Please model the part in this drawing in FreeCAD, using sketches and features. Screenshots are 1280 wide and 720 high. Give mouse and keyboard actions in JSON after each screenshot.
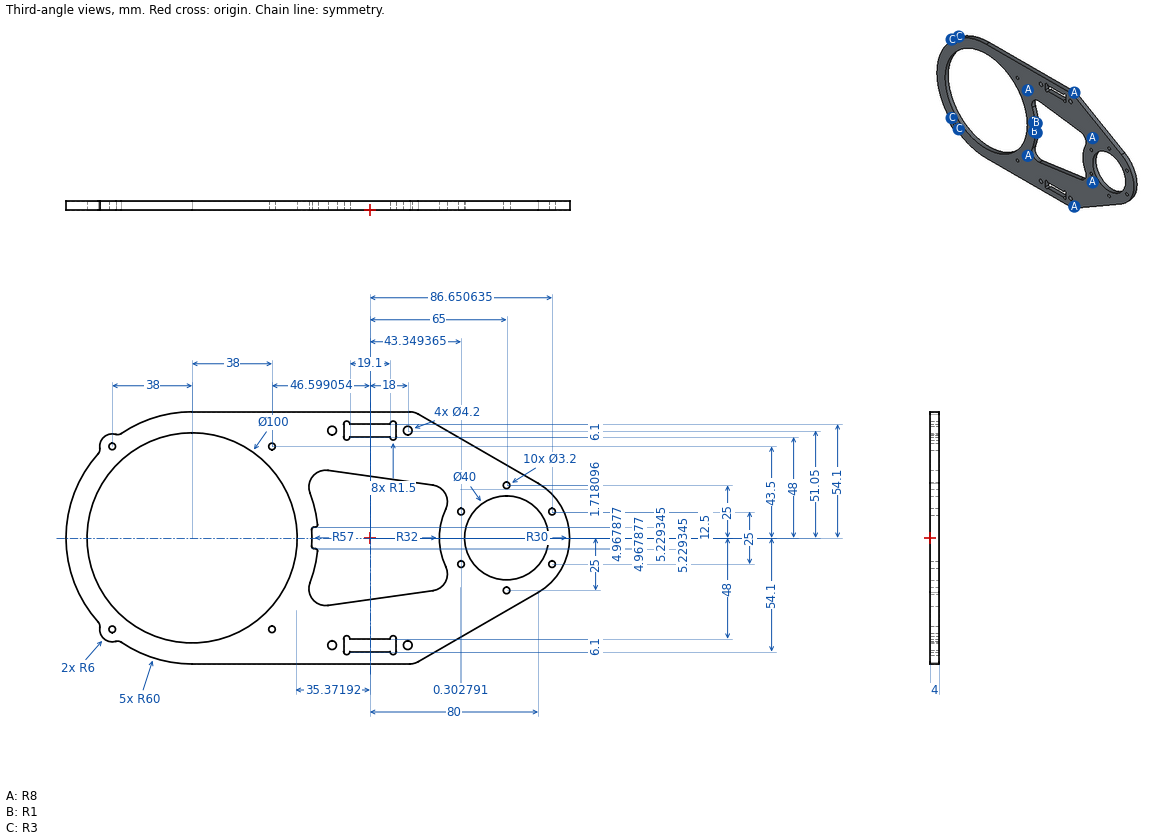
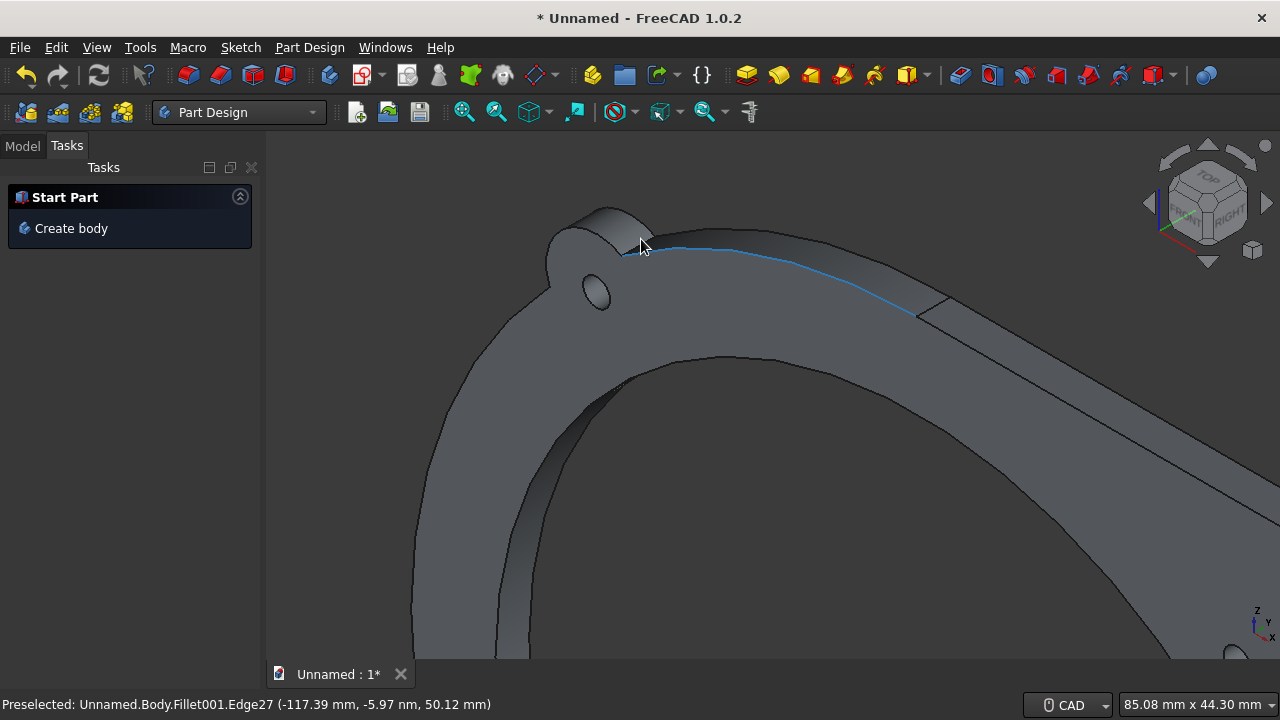
{"action": "left_click", "coordinate": [466, 112]}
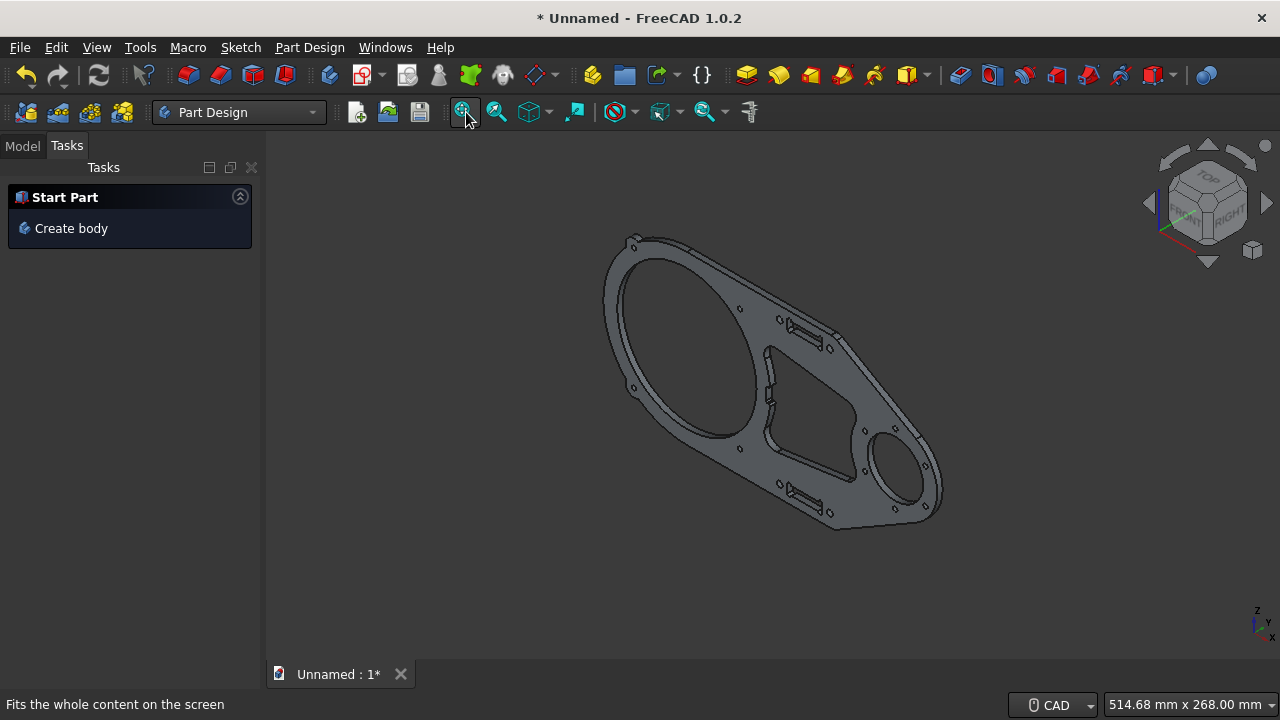
{"action": "key", "text": "2"}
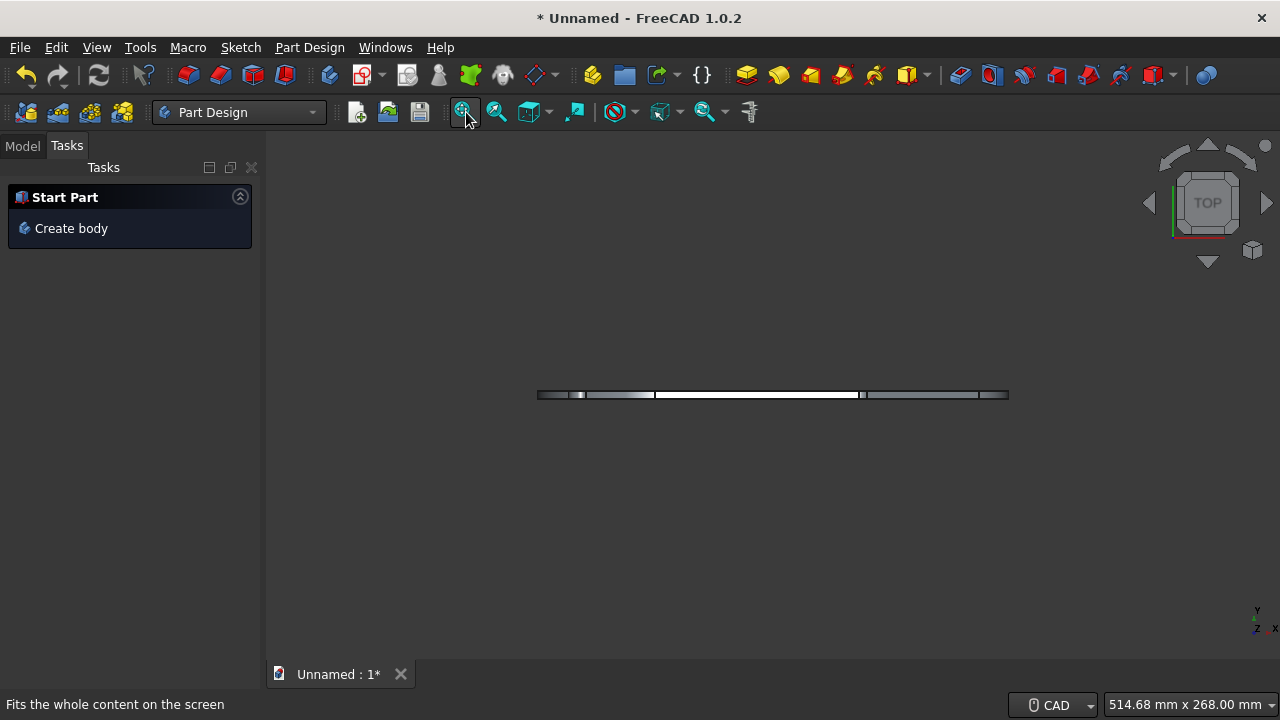
{"action": "scroll", "coordinate": [586, 394], "scroll_direction": "up", "scroll_amount": 9}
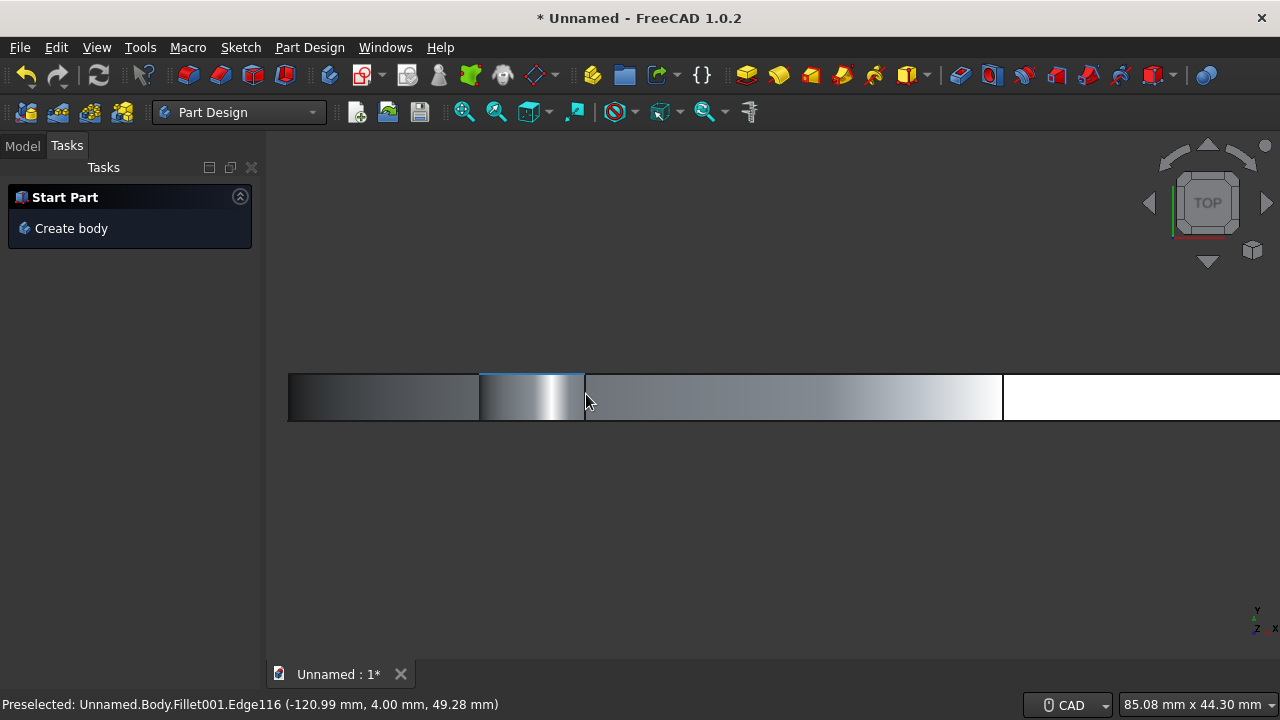
{"action": "left_click", "coordinate": [466, 112]}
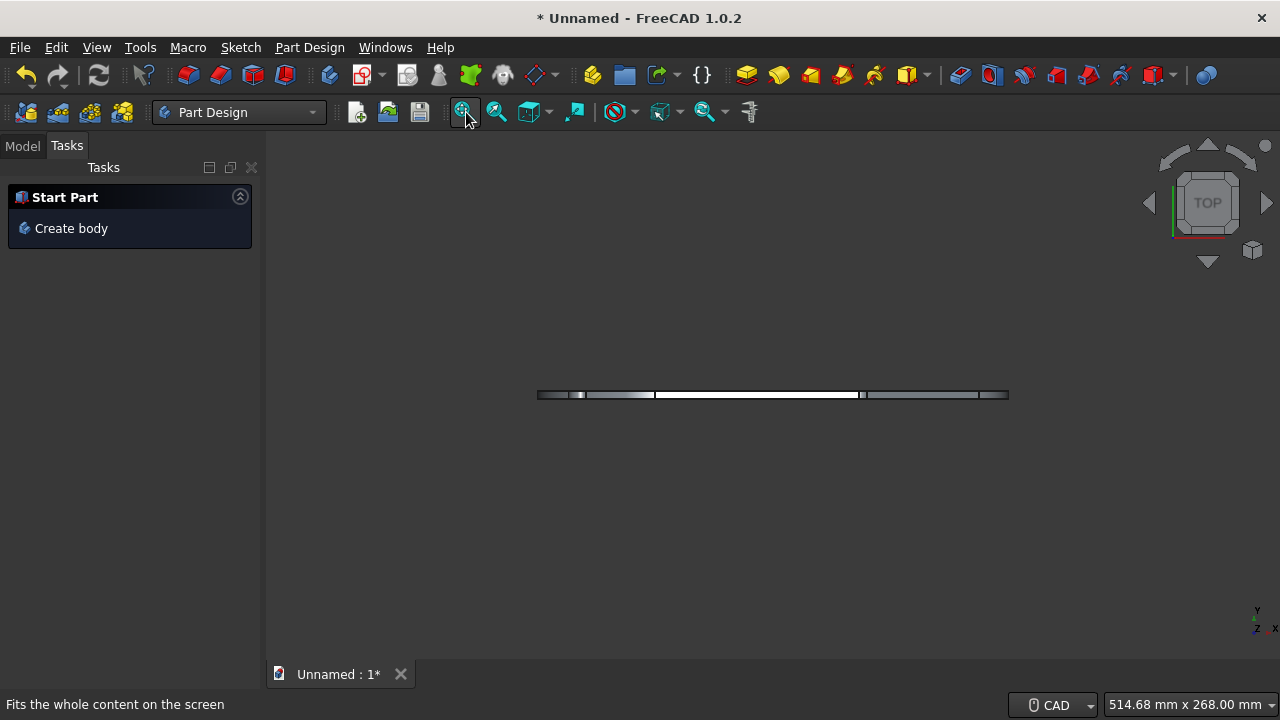
{"action": "key", "text": "0"}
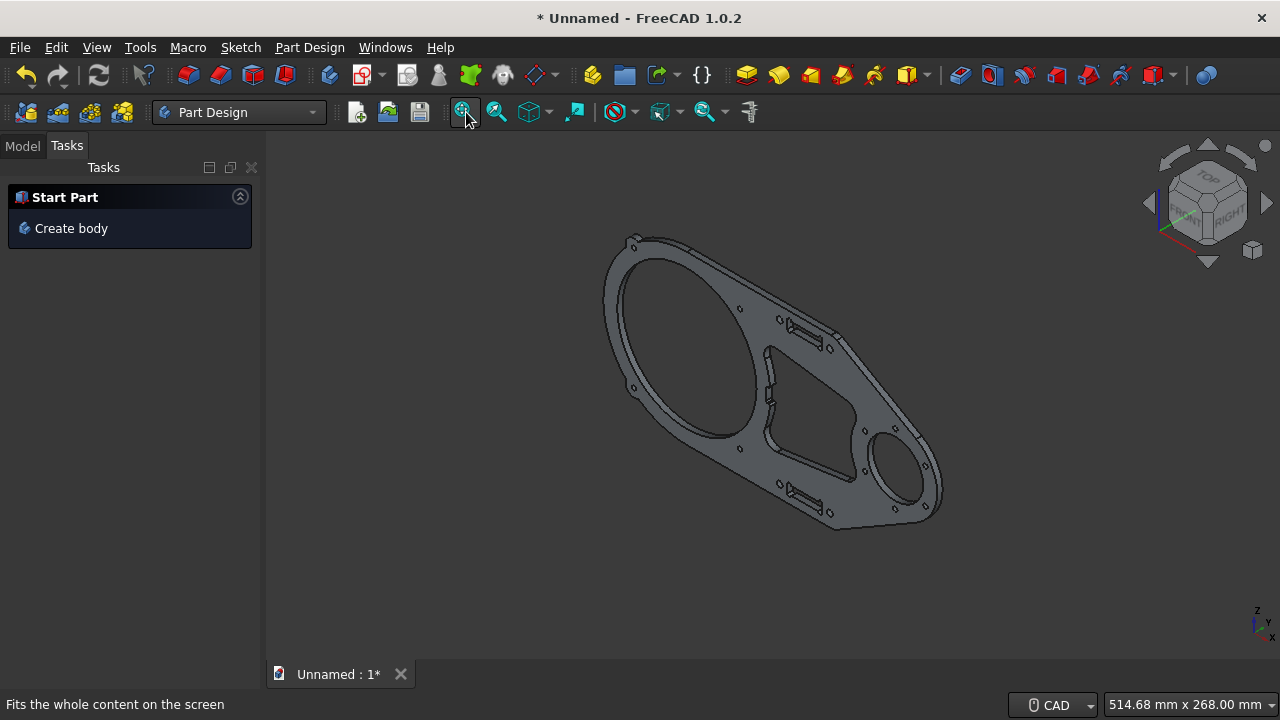
{"action": "scroll", "coordinate": [641, 239], "scroll_direction": "up", "scroll_amount": 9}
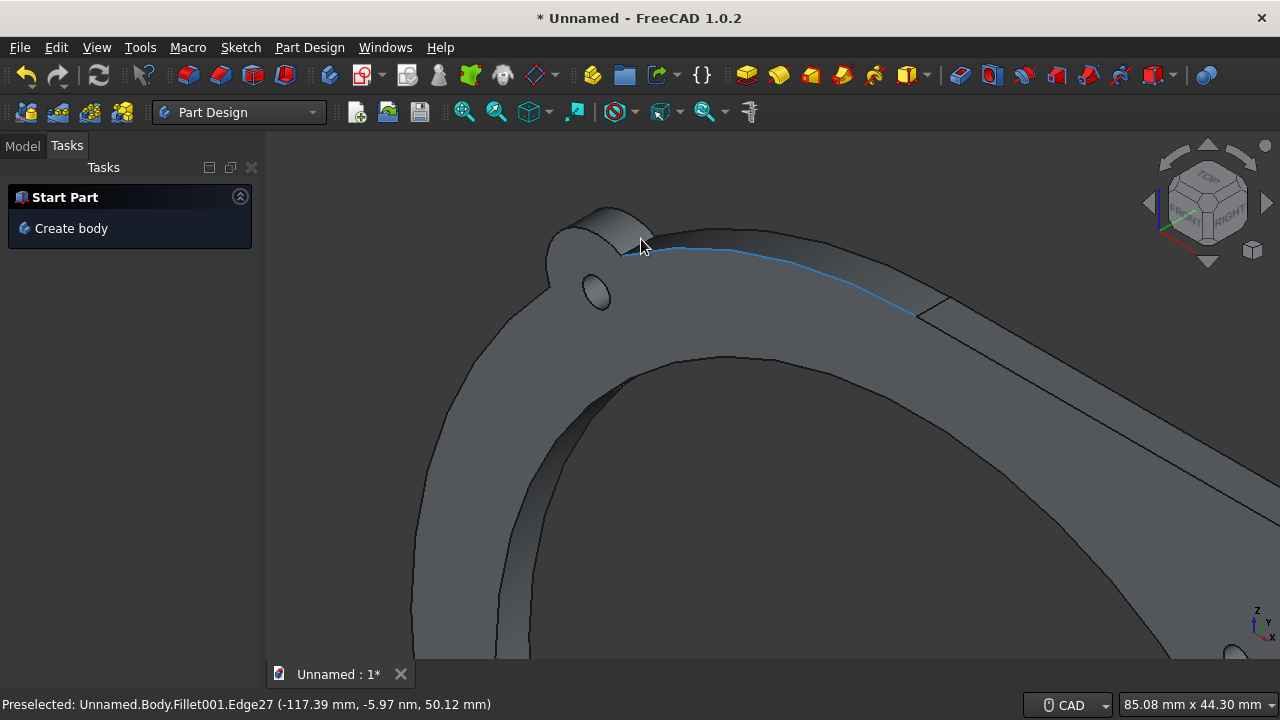
{"action": "key", "text": "v f"}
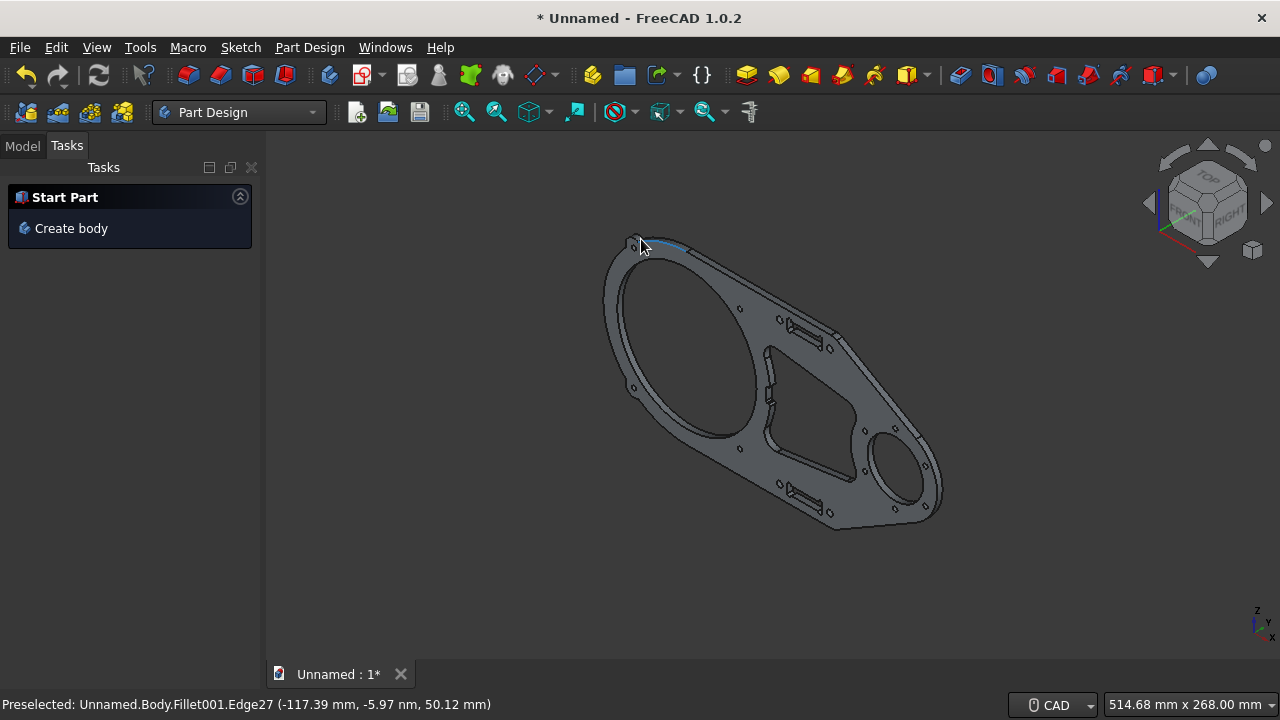
{"action": "key", "text": "1"}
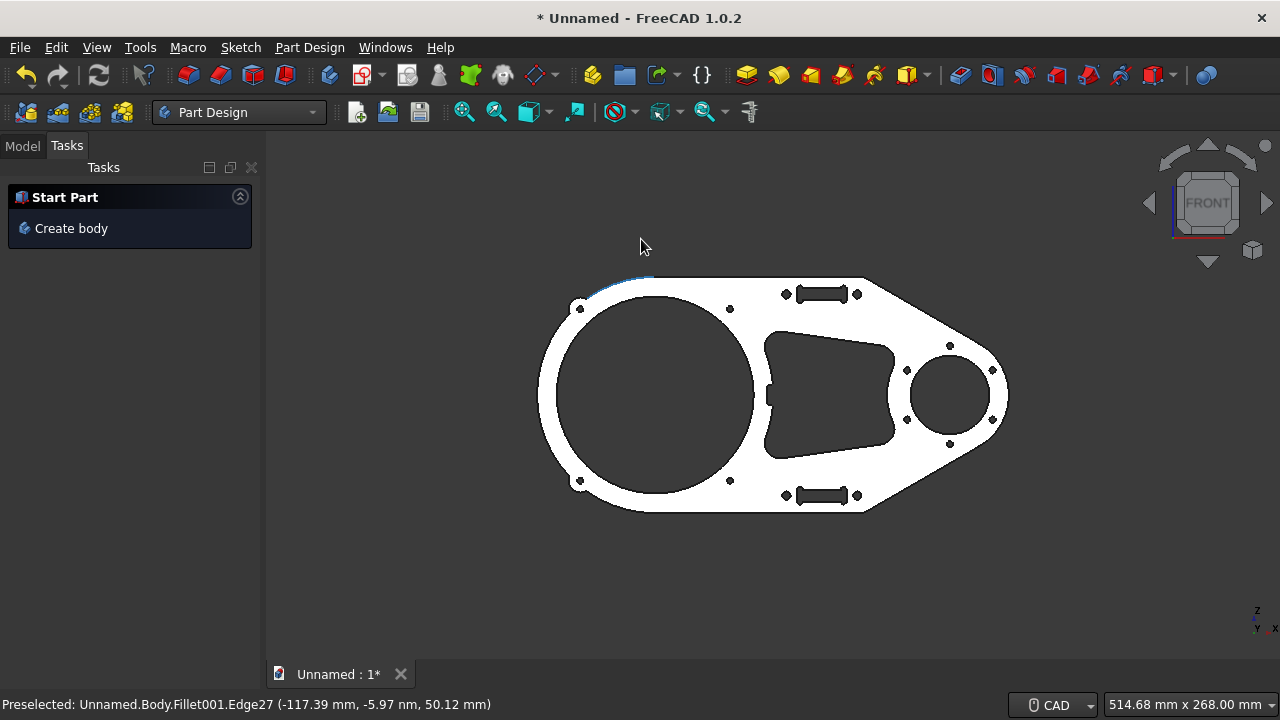
{"action": "scroll", "coordinate": [586, 298], "scroll_direction": "up", "scroll_amount": 9}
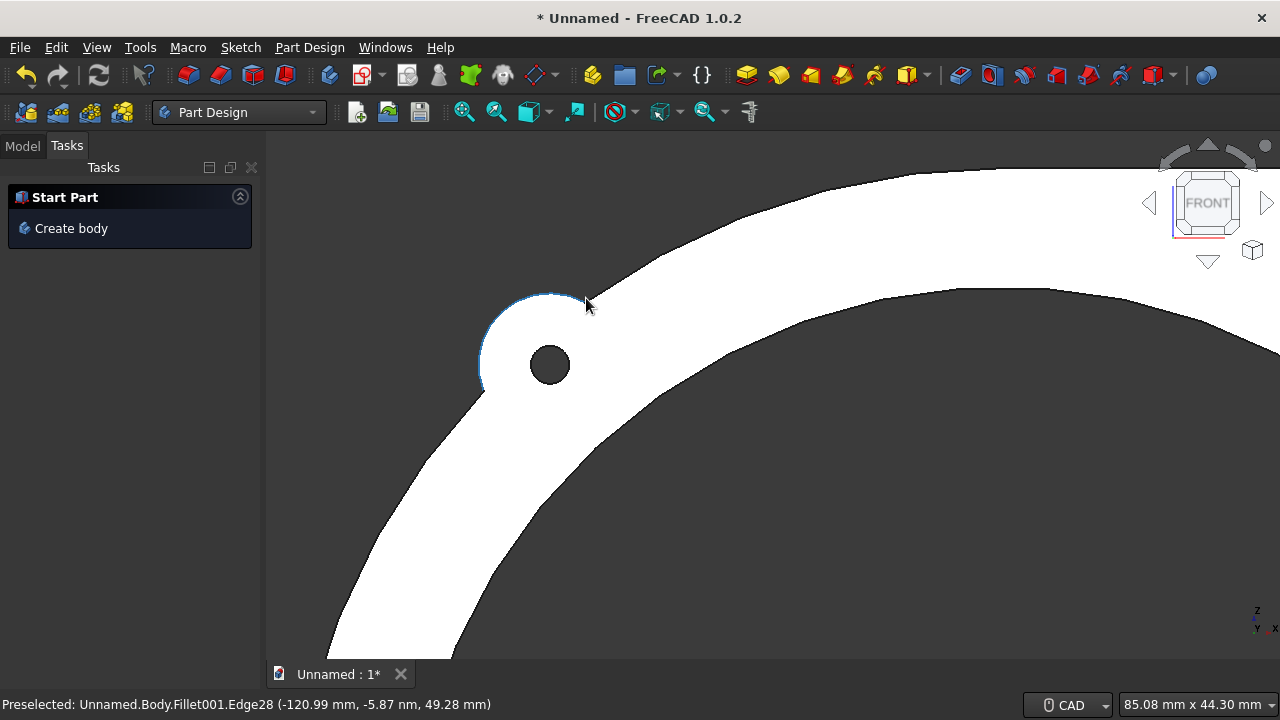
{"action": "left_click", "coordinate": [466, 112]}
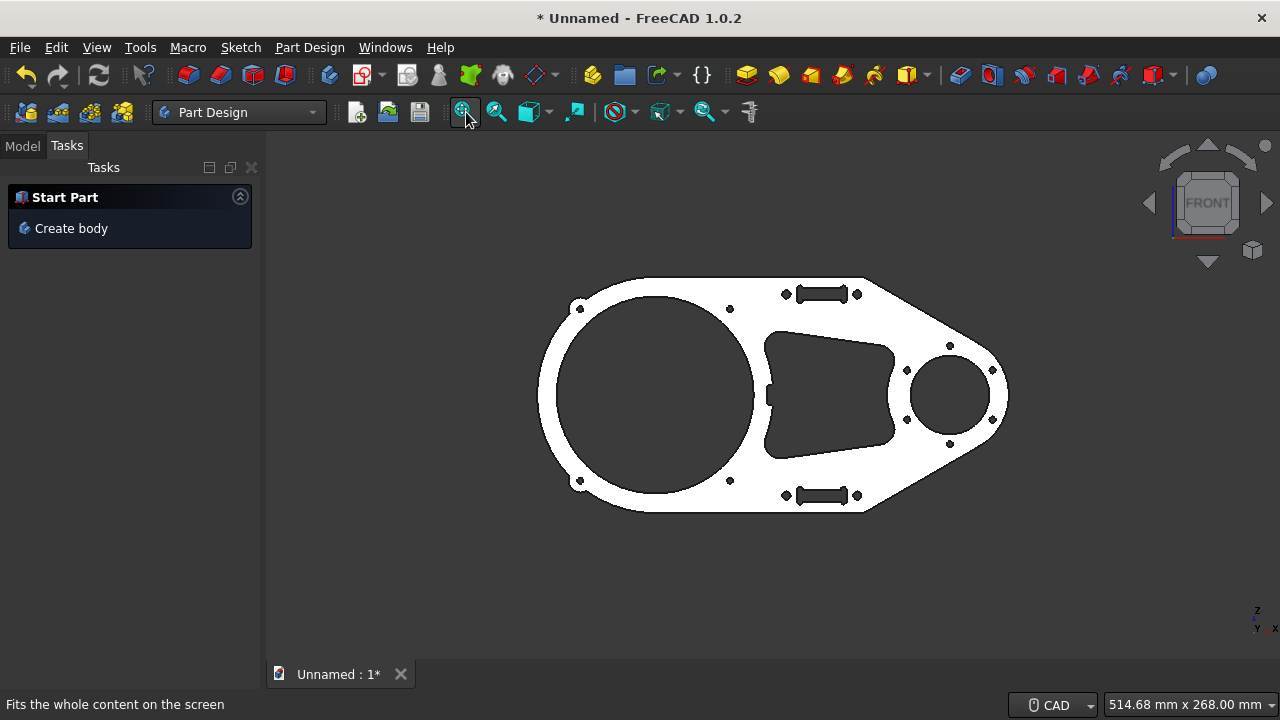
{"action": "key", "text": "3"}